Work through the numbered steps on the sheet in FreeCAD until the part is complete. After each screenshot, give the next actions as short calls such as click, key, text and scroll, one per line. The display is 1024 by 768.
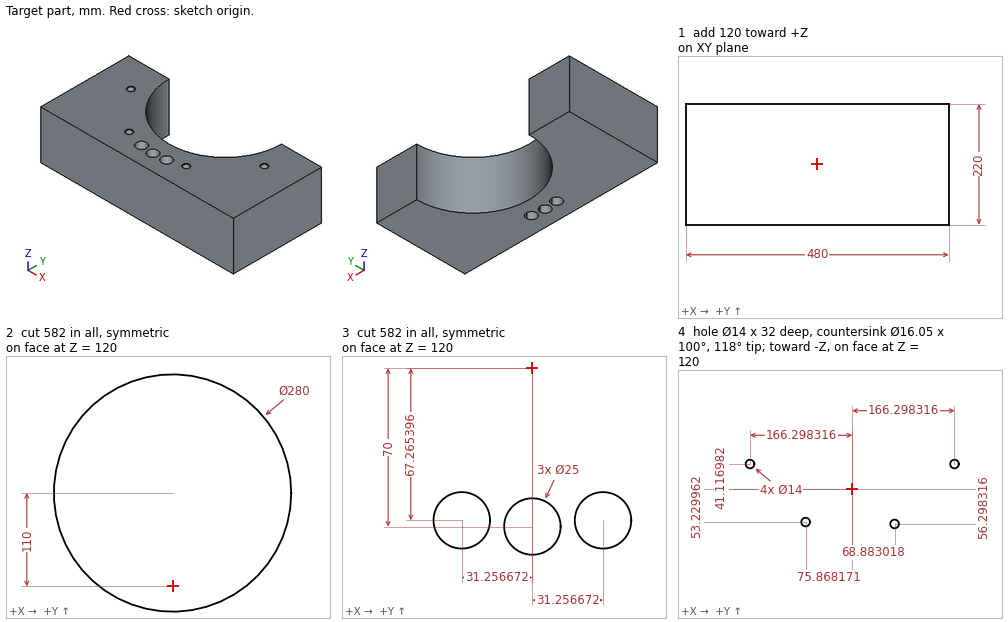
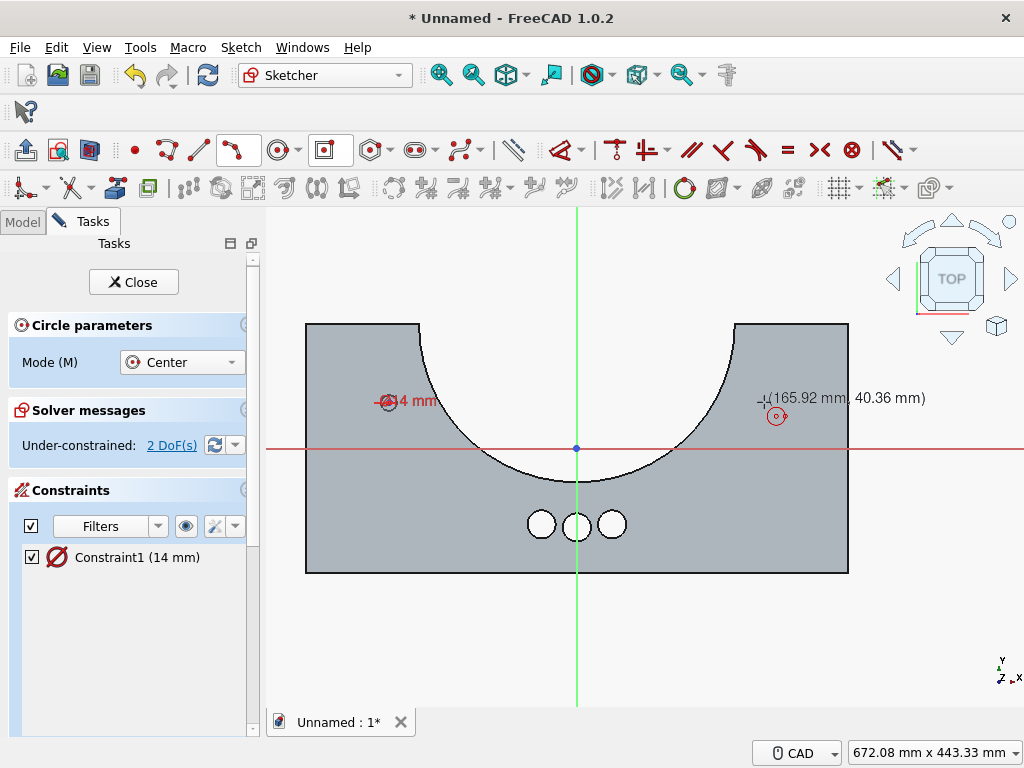
click(764, 402)
move(770, 397)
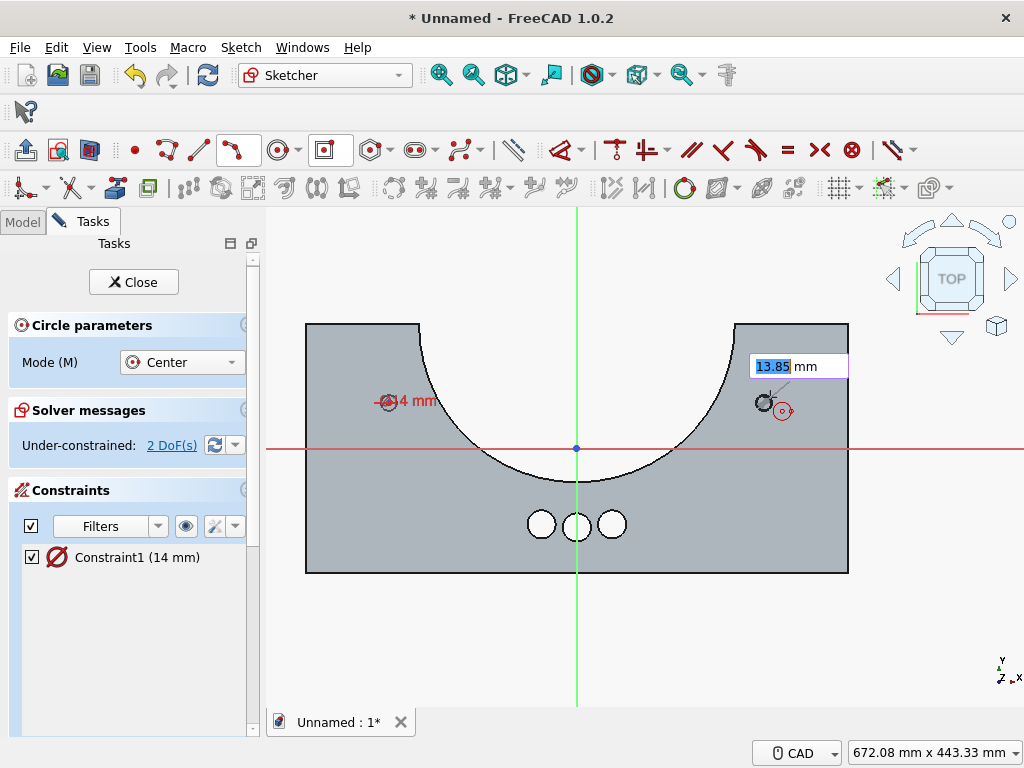
text(14)
key(Return)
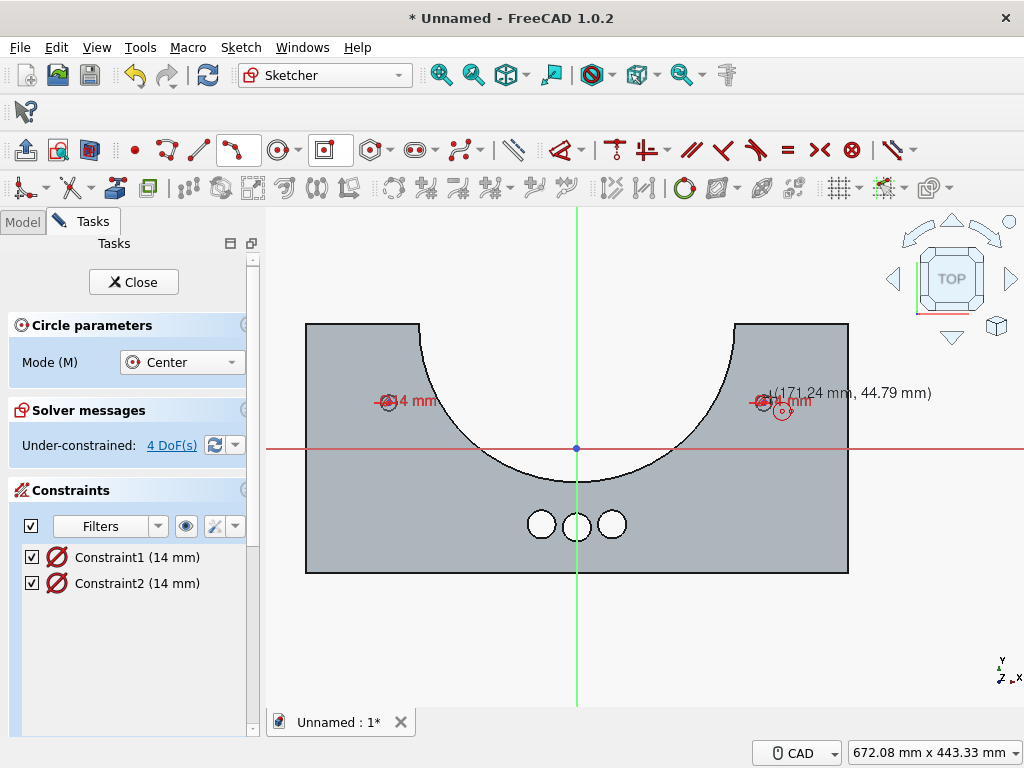
scroll(655, 512, up, 6)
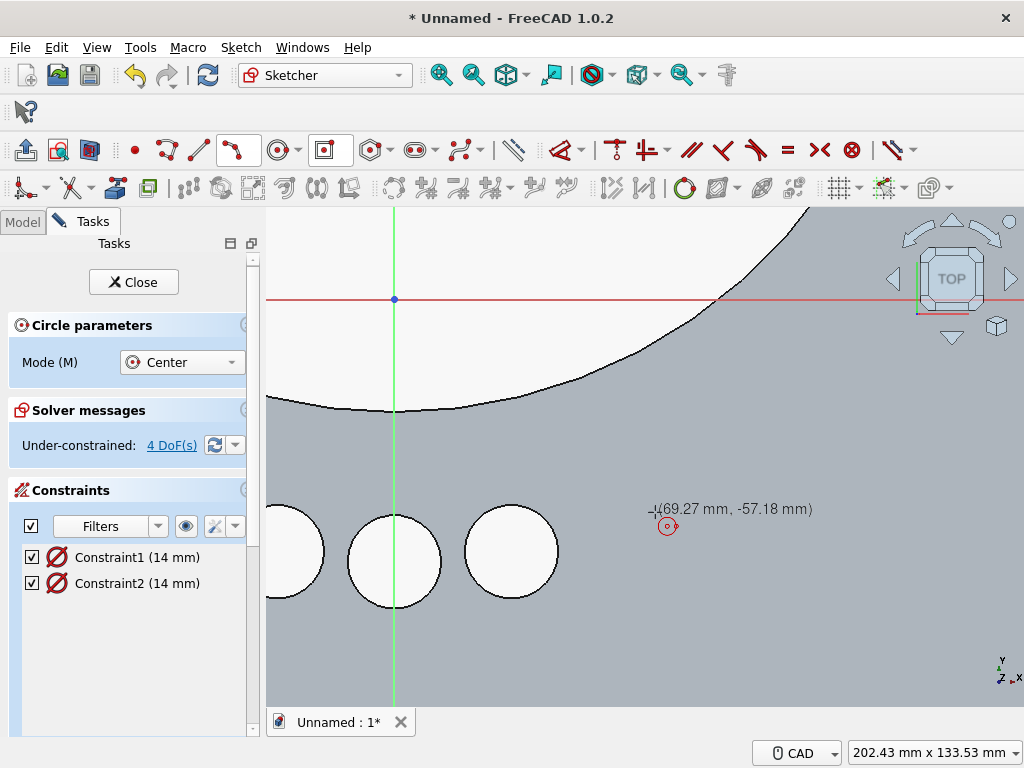
scroll(655, 513, down, 6)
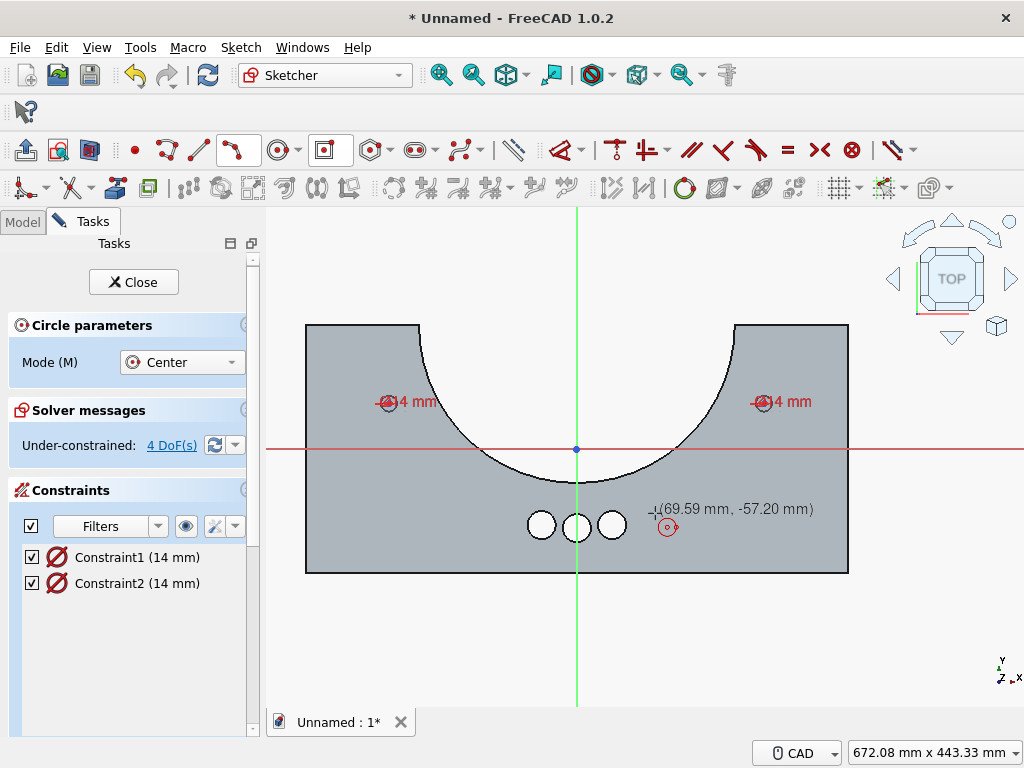
click(655, 513)
move(660, 507)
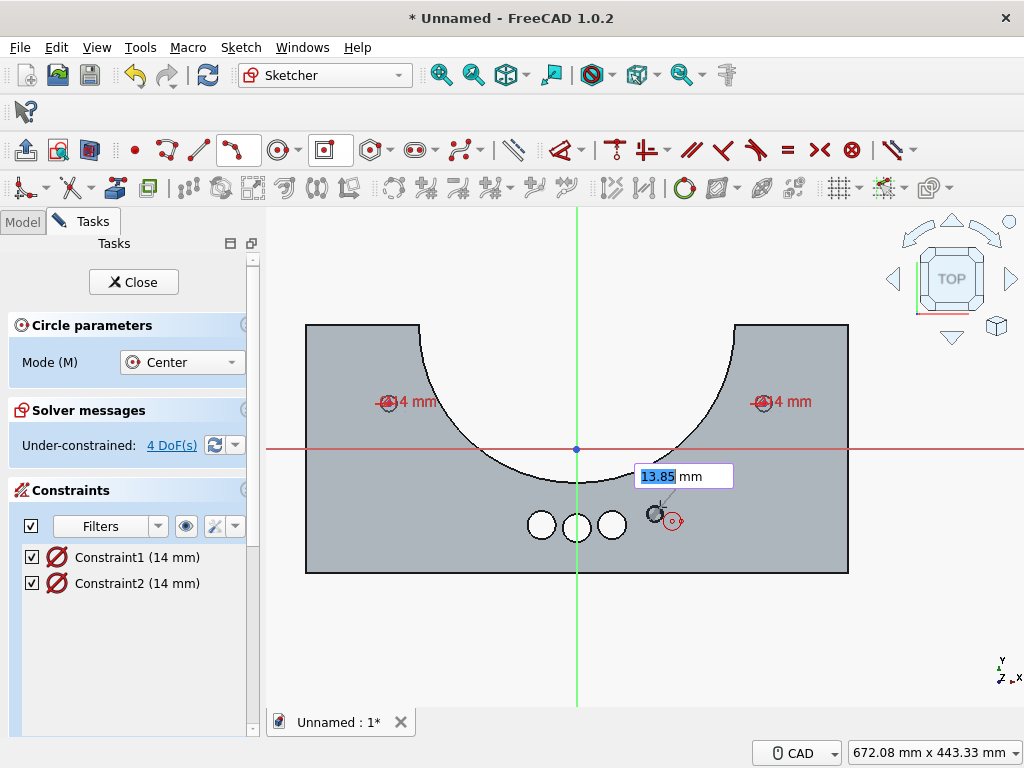
text(14)
key(Return)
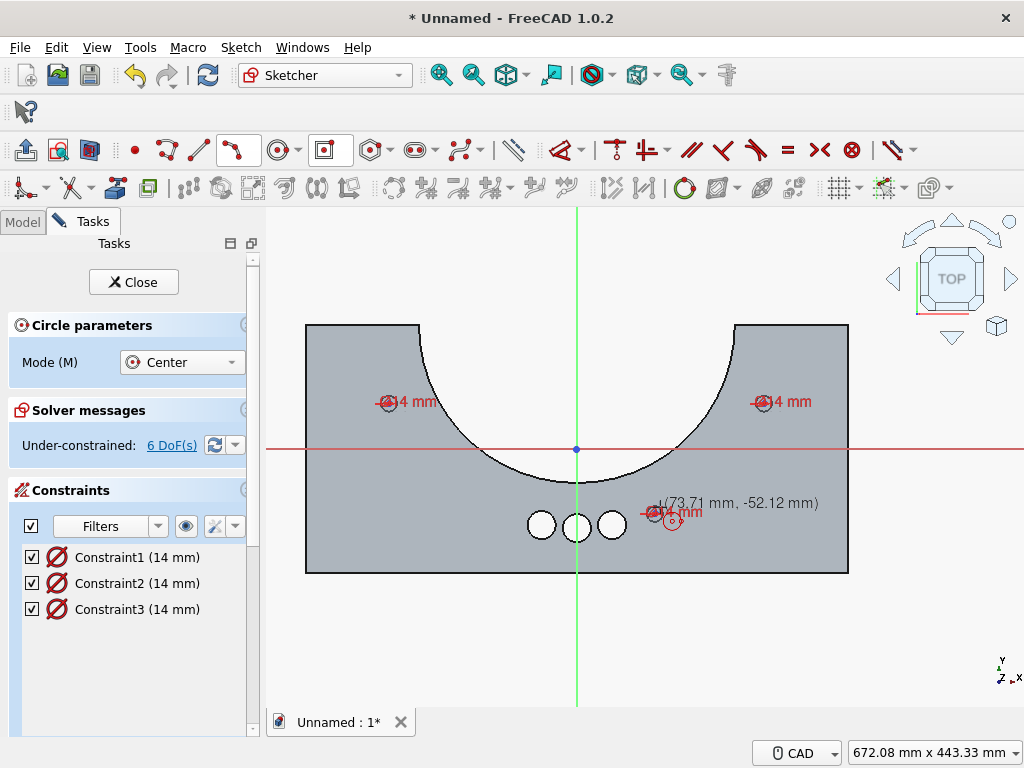
scroll(491, 509, up, 6)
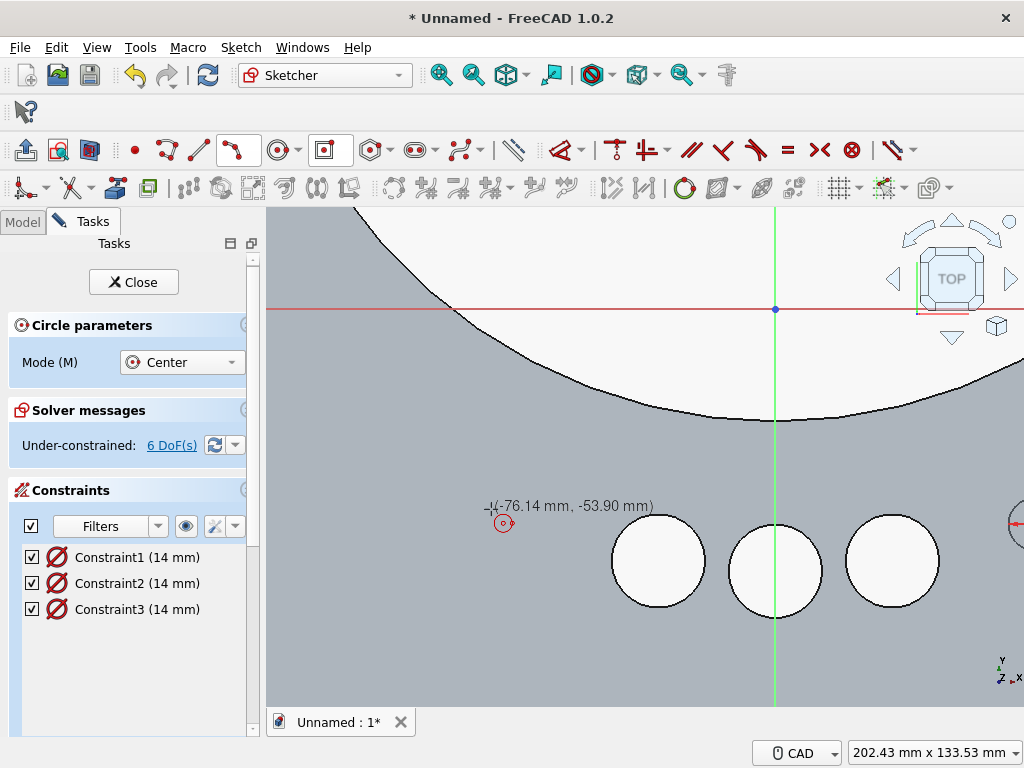
scroll(491, 508, down, 6)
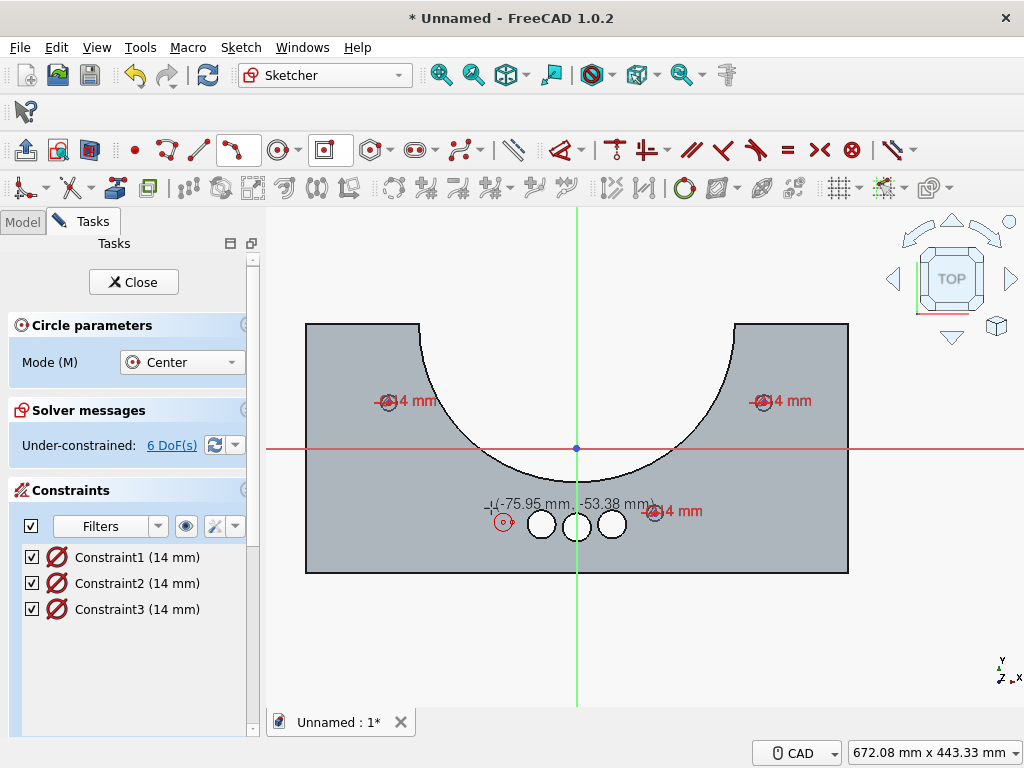
click(491, 509)
move(497, 503)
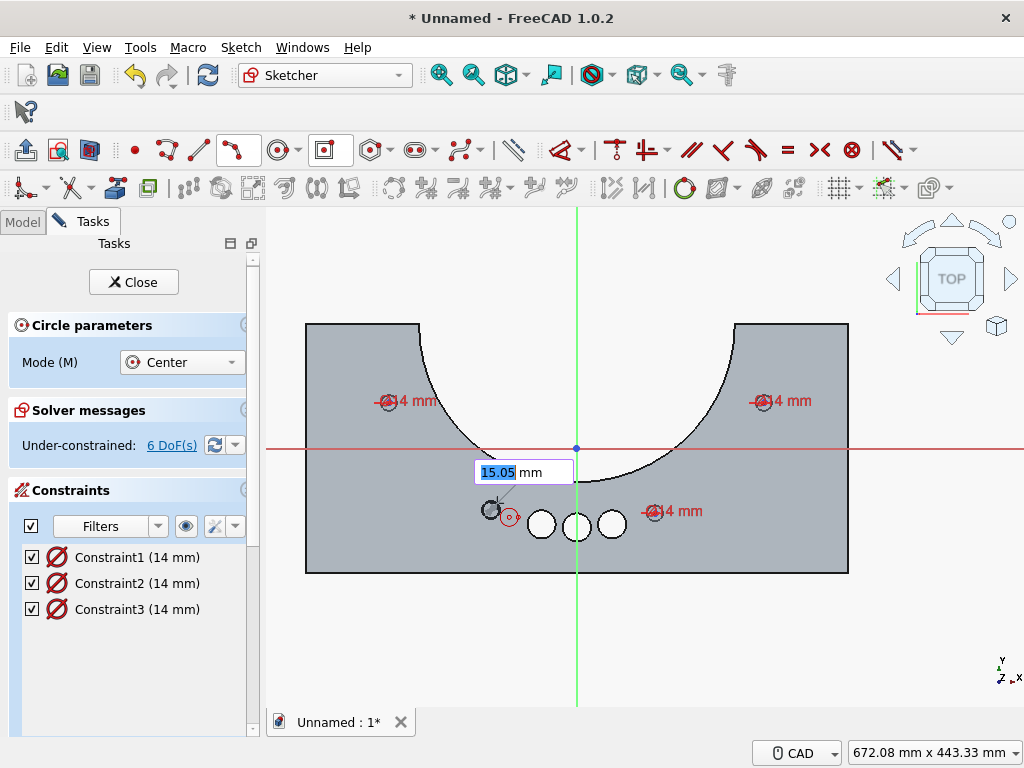
text(14)
key(Return)
key(Escape)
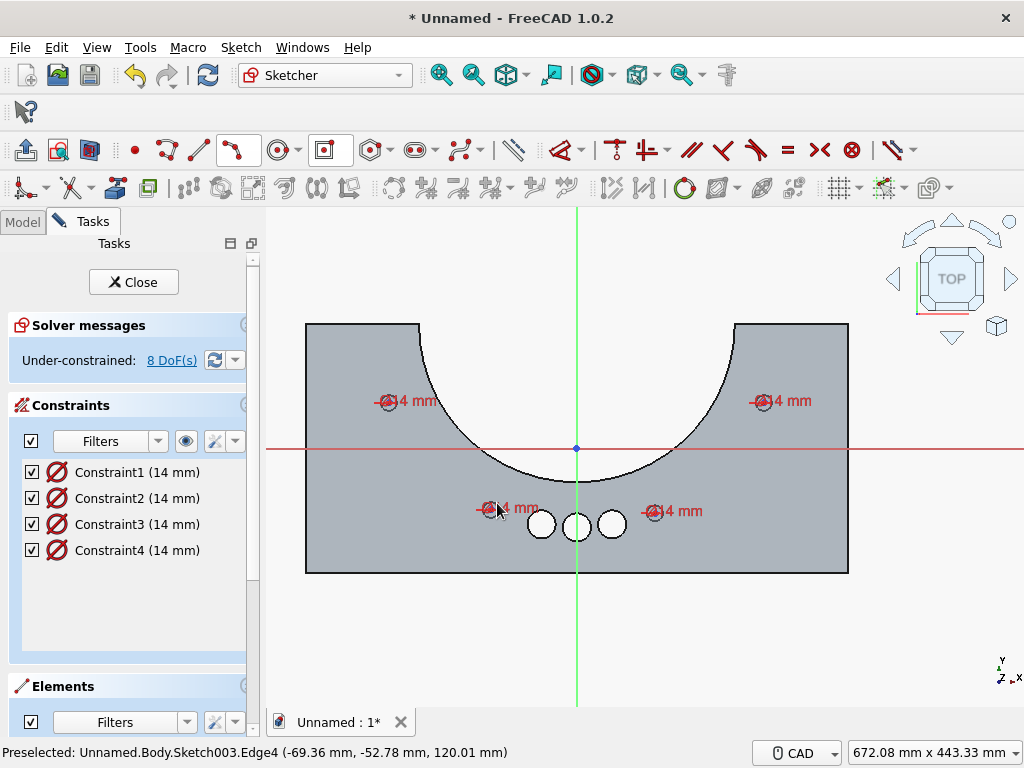
click(389, 403)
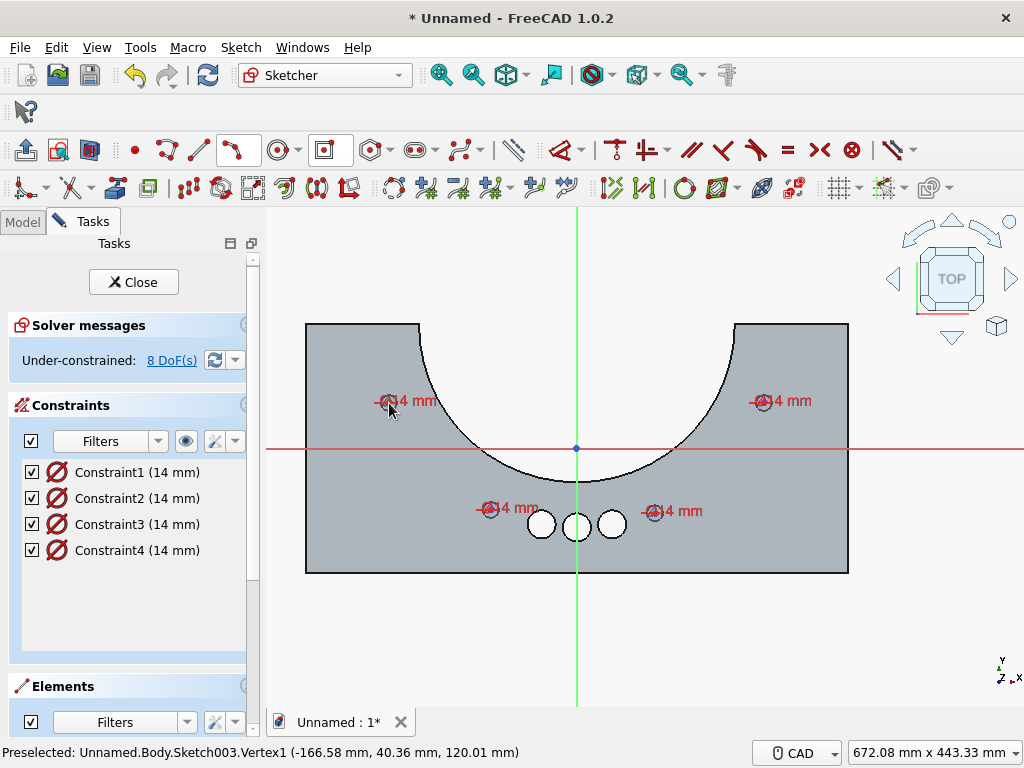
click(764, 403)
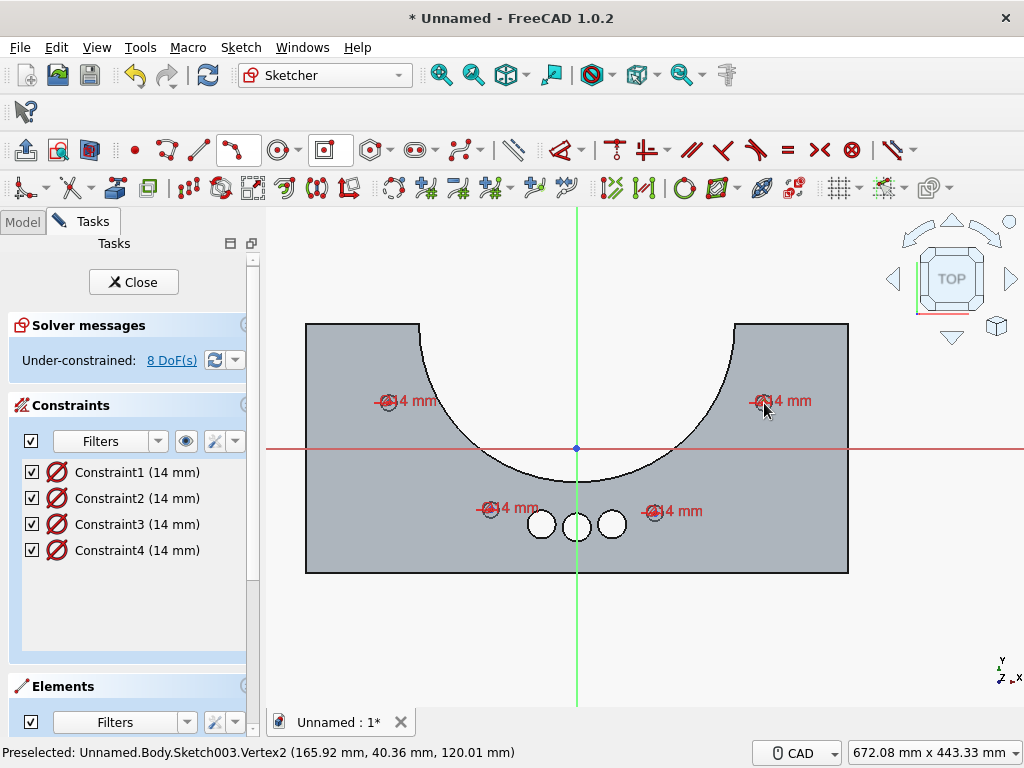
key(h)